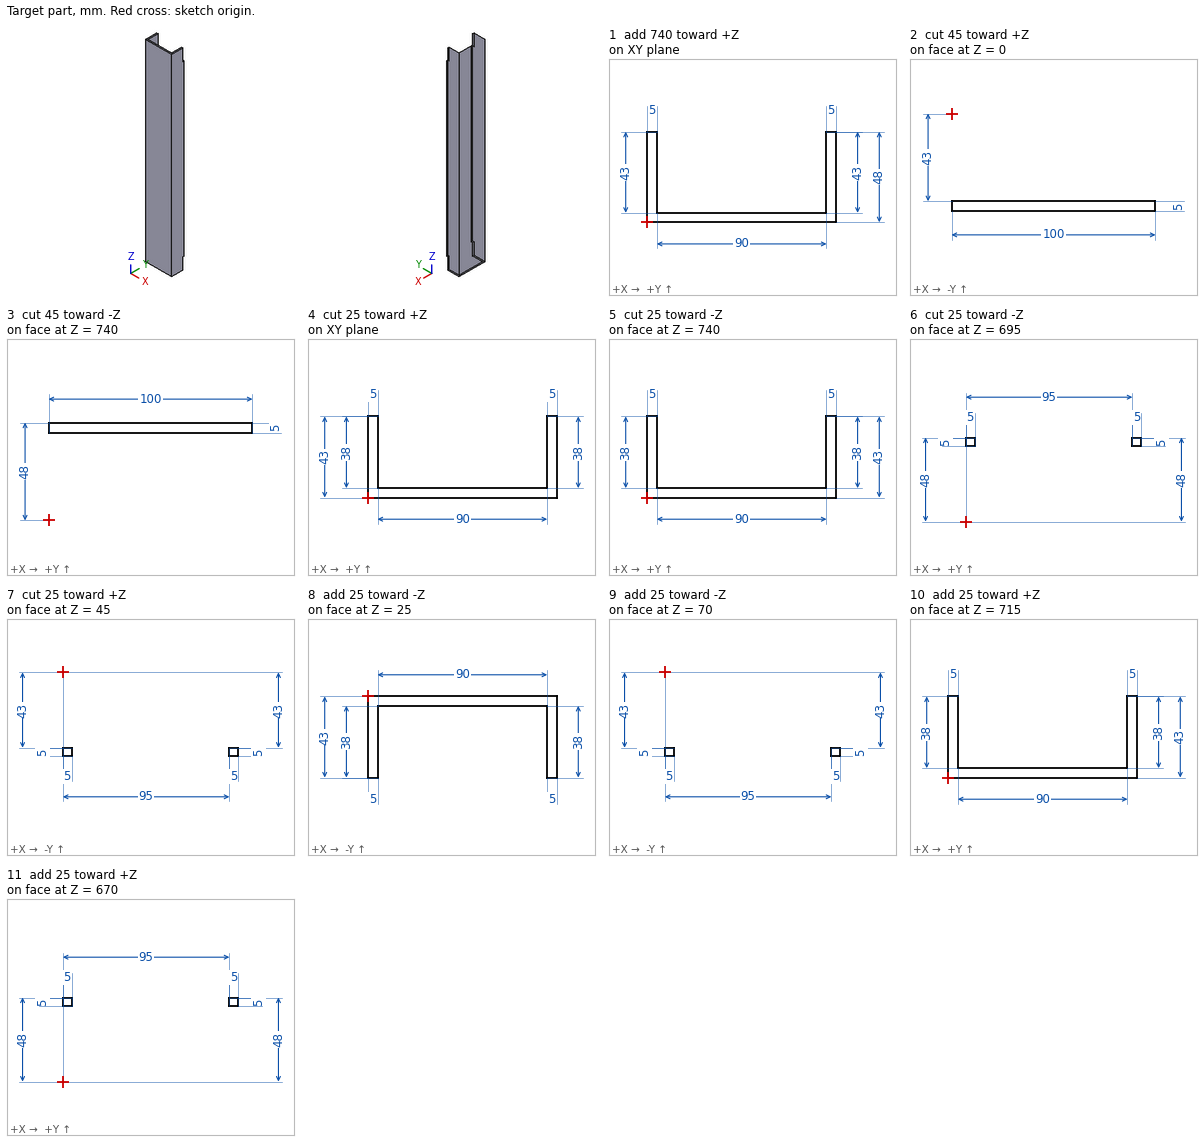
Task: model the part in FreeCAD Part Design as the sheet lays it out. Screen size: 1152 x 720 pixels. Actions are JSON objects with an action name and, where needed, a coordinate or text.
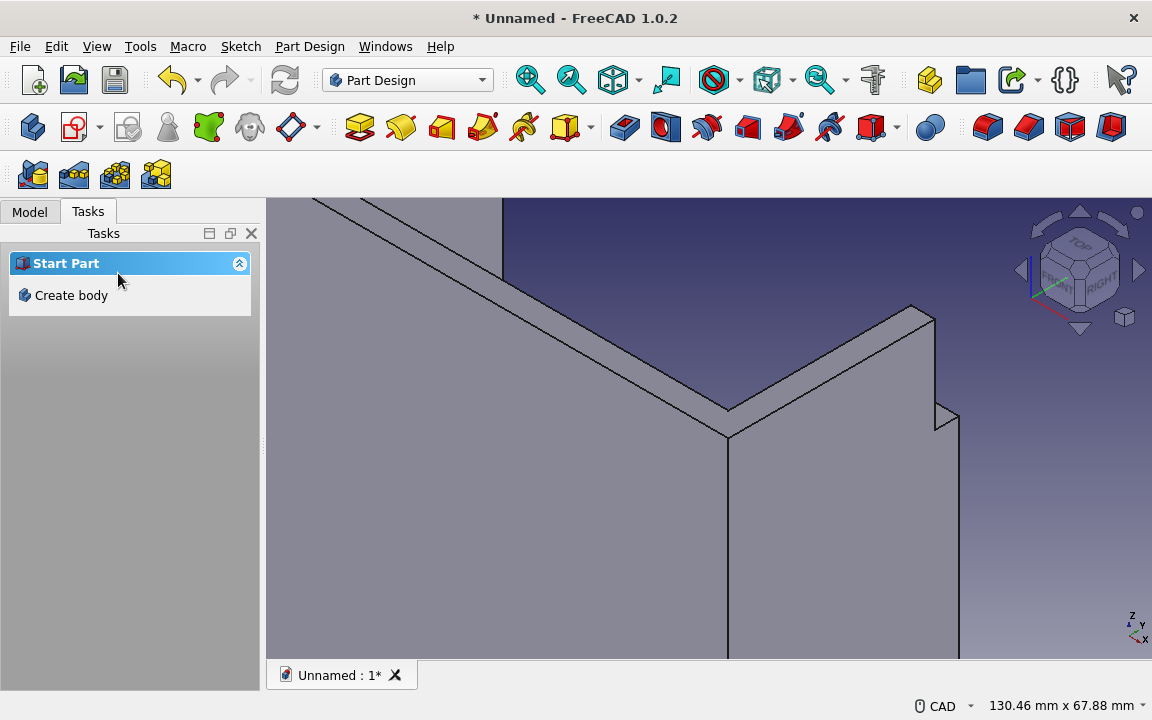
{"action": "left_click", "coordinate": [531, 80]}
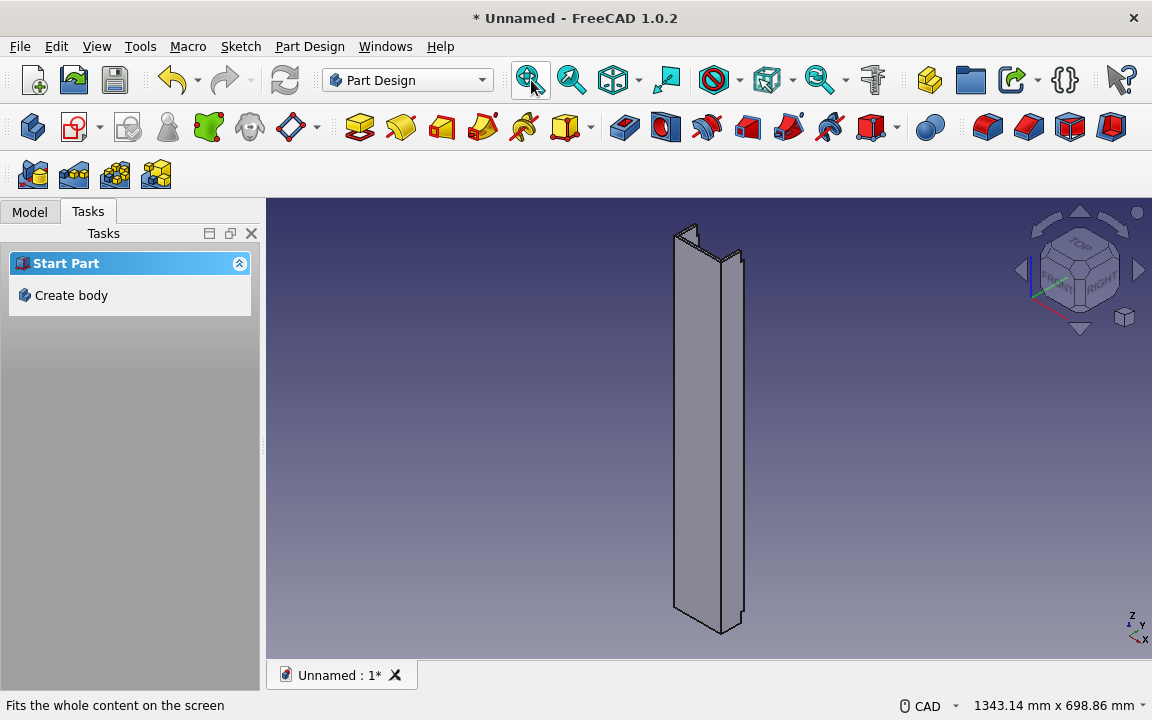
{"action": "scroll", "coordinate": [741, 259], "scroll_direction": "up", "scroll_amount": 10}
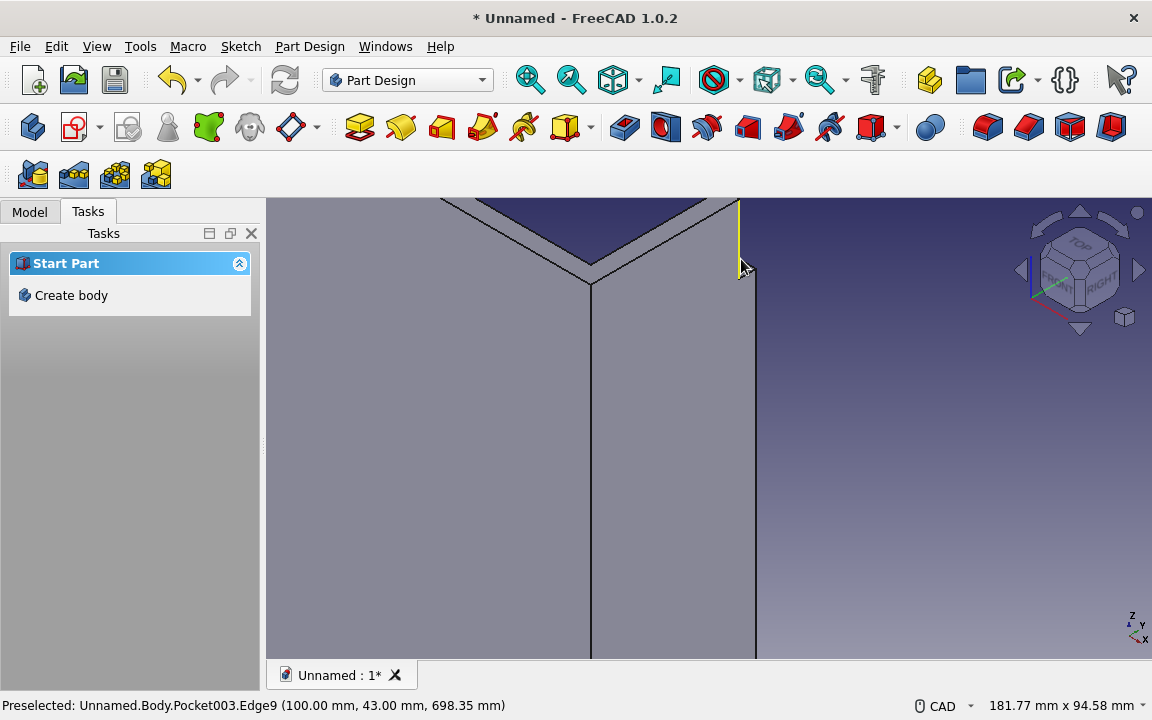
{"action": "left_click", "coordinate": [531, 80]}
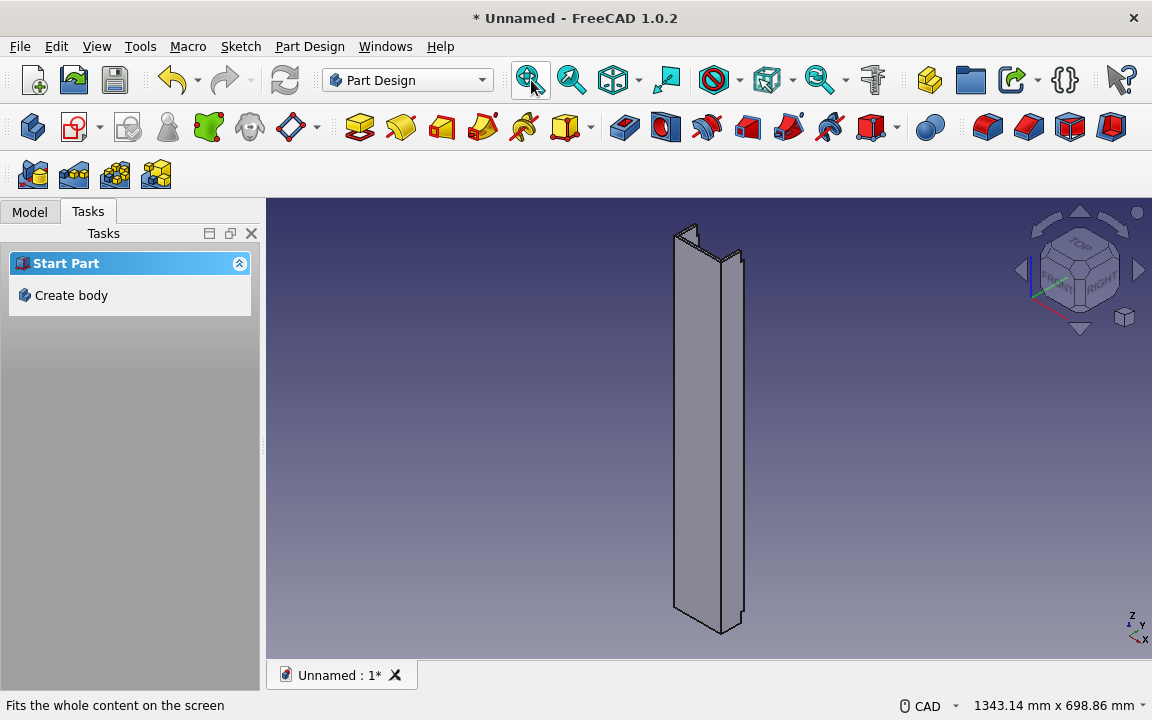
{"action": "key", "text": "2"}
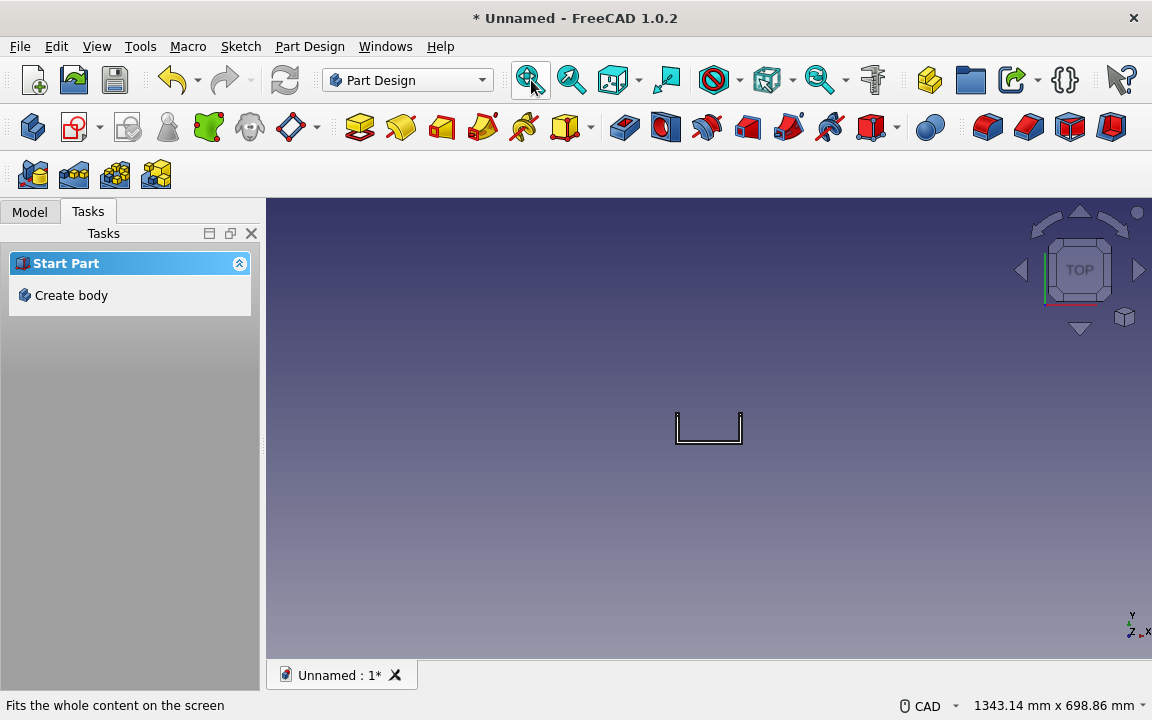
{"action": "key", "text": "v f"}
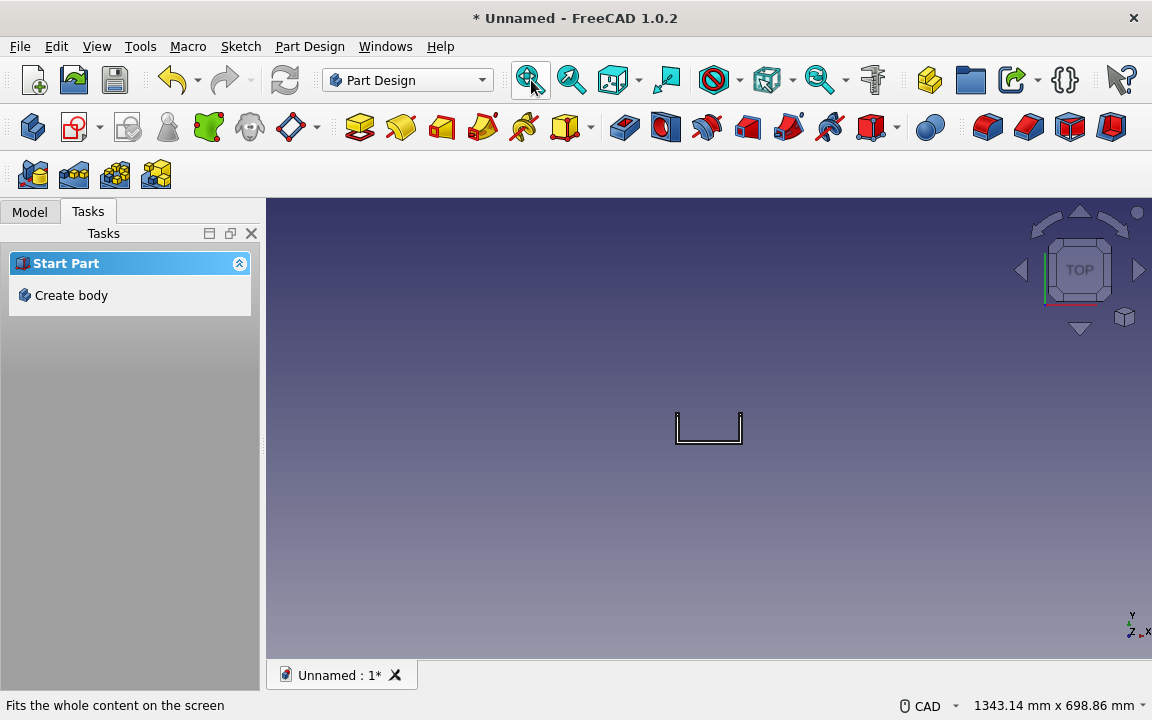
{"action": "scroll", "coordinate": [740, 413], "scroll_direction": "up", "scroll_amount": 10}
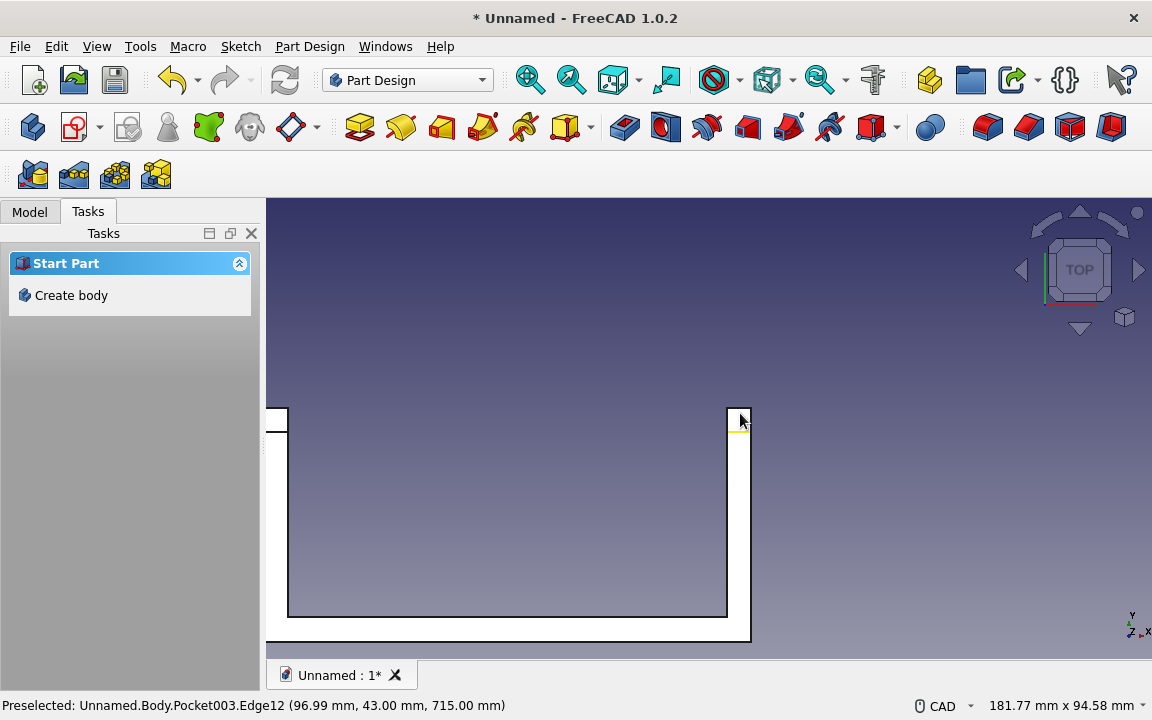
{"action": "left_click", "coordinate": [739, 419]}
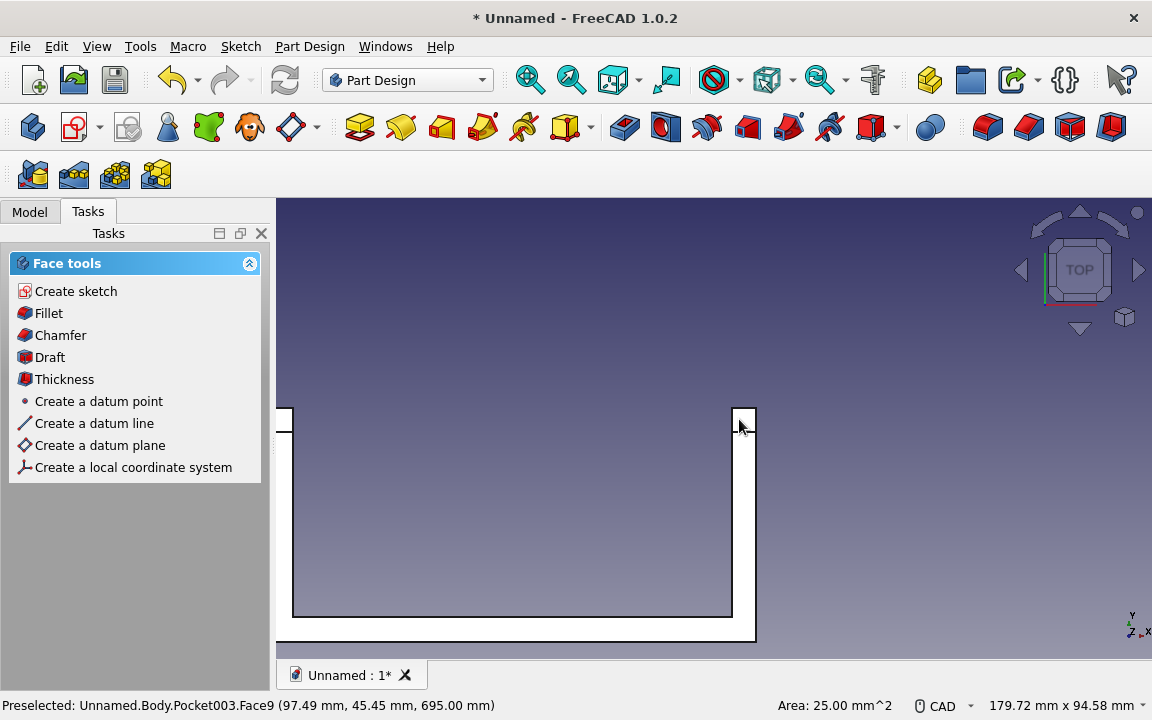
{"action": "left_click", "coordinate": [74, 128]}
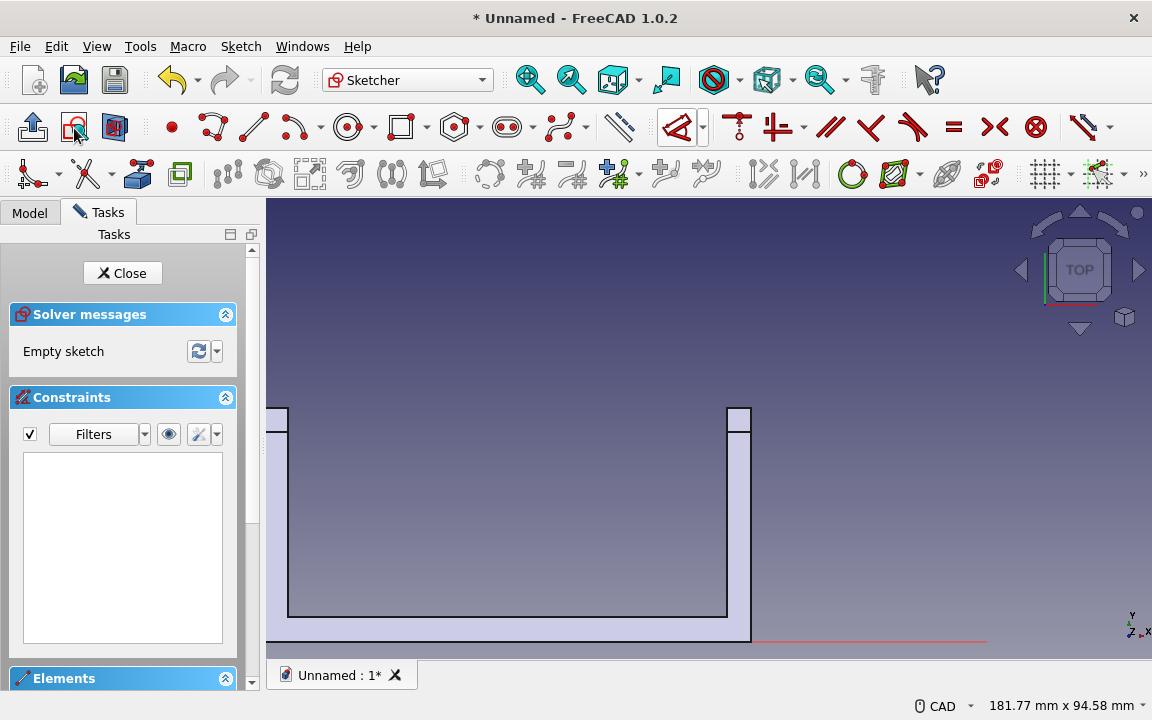
{"action": "scroll", "coordinate": [987, 226], "scroll_direction": "down", "scroll_amount": 1}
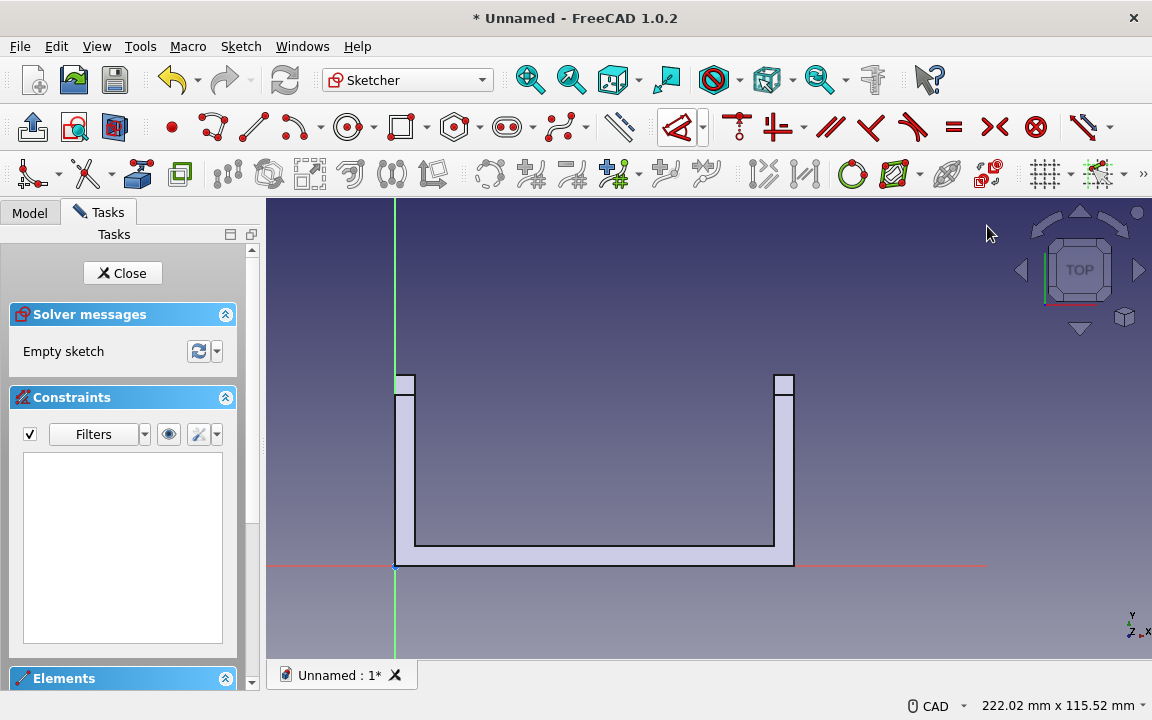
{"action": "key", "text": "g r"}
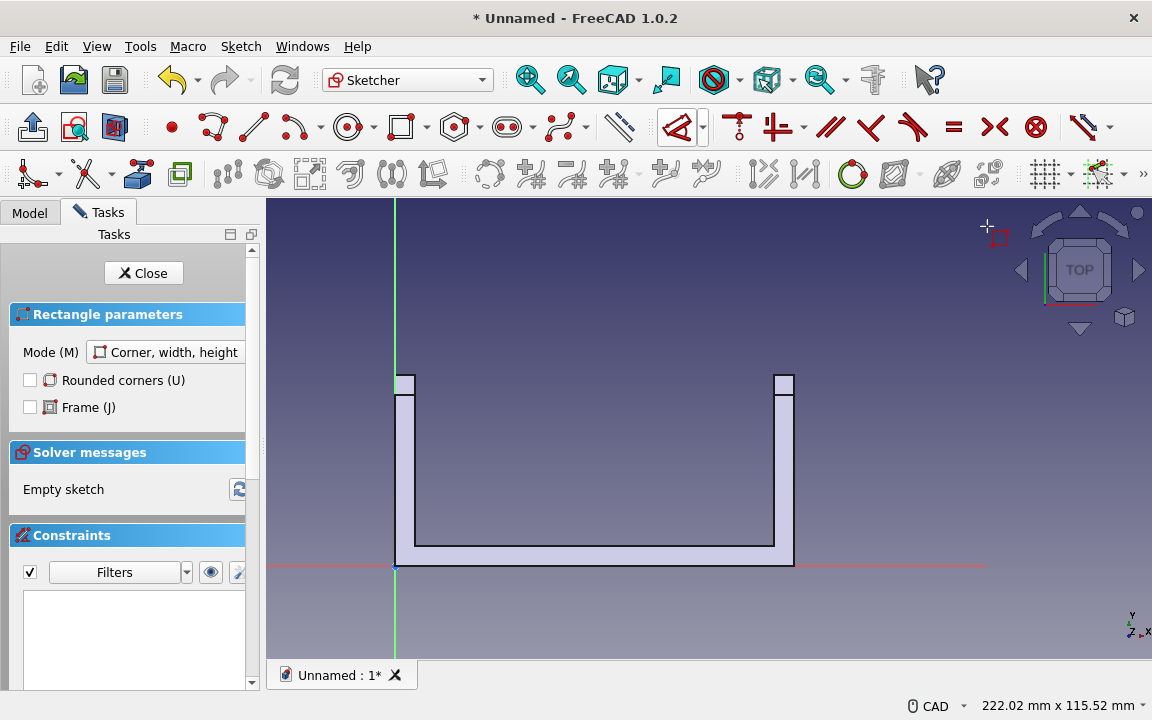
{"action": "left_click", "coordinate": [774, 375]}
{"action": "mouse_move", "coordinate": [794, 395]}